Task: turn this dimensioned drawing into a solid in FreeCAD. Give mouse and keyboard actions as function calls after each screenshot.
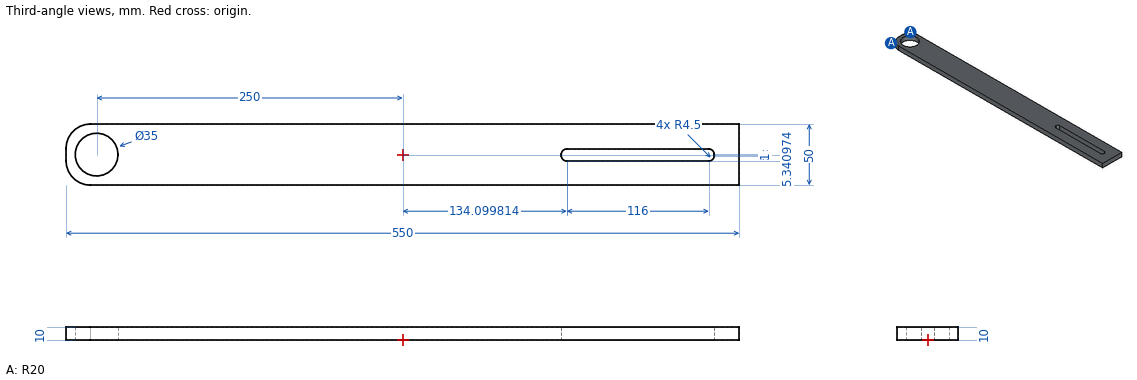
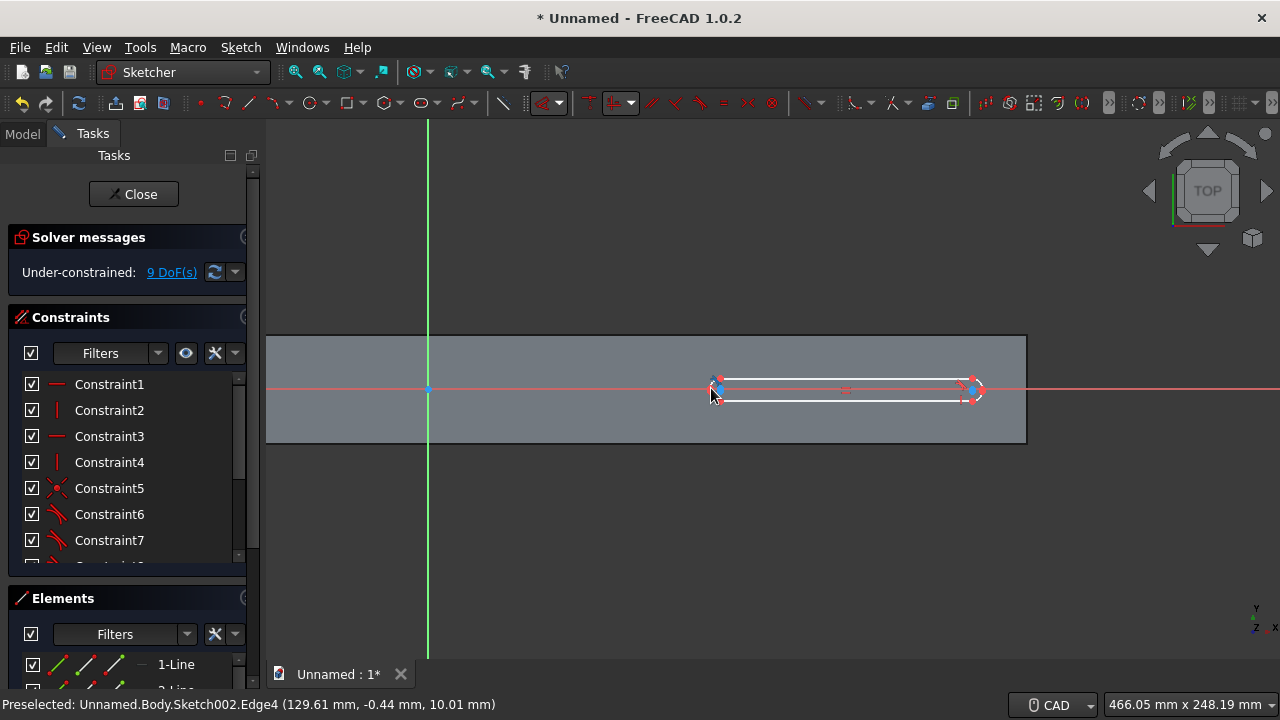
scroll(711, 396, up, 6)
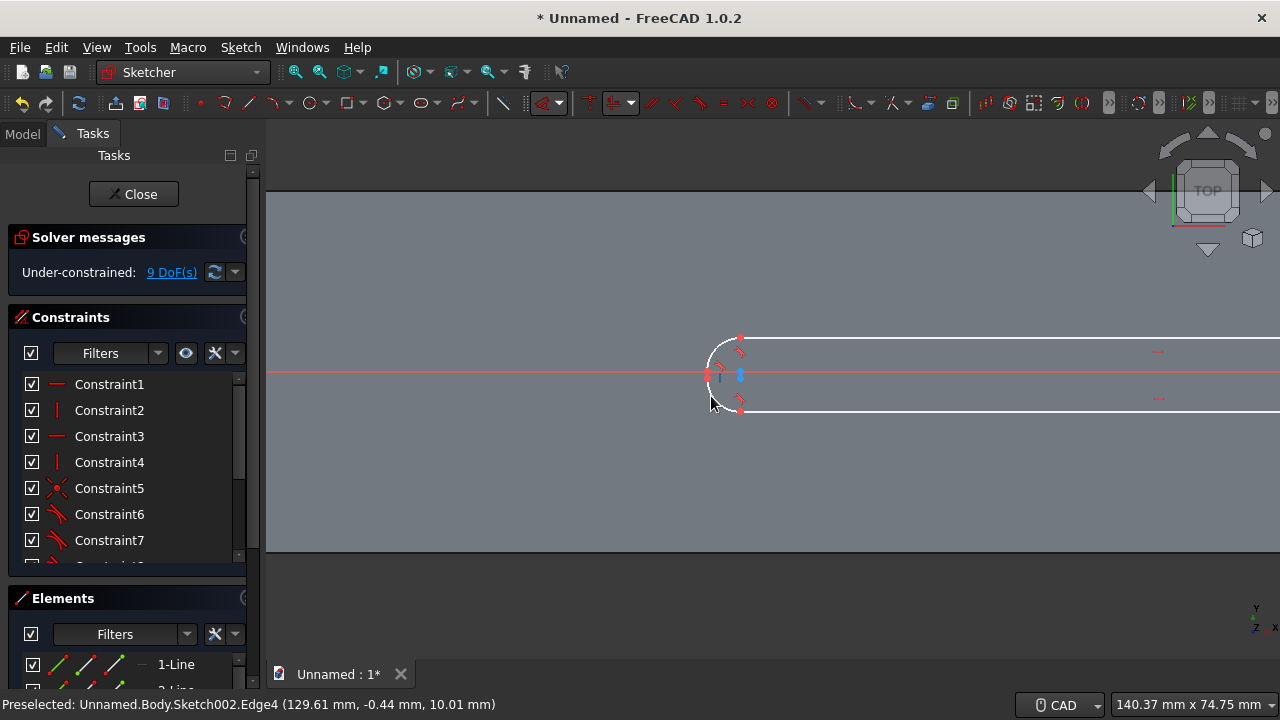
click(711, 394)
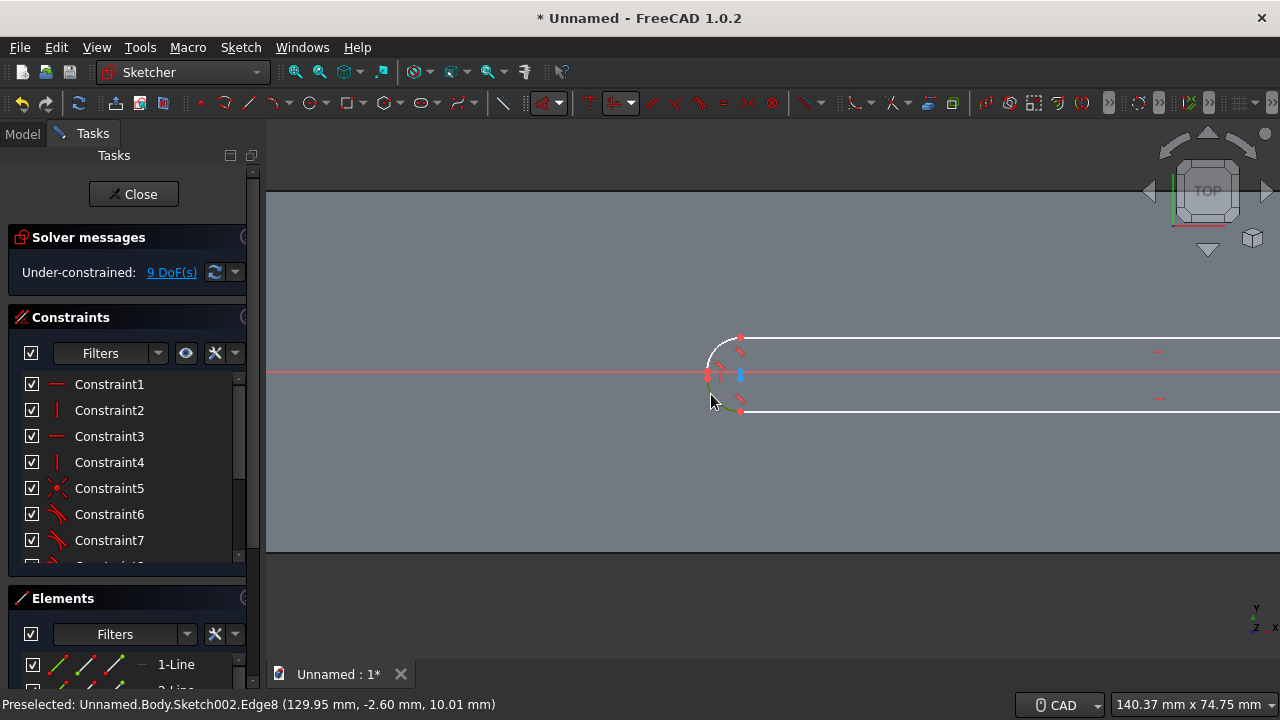
click(700, 104)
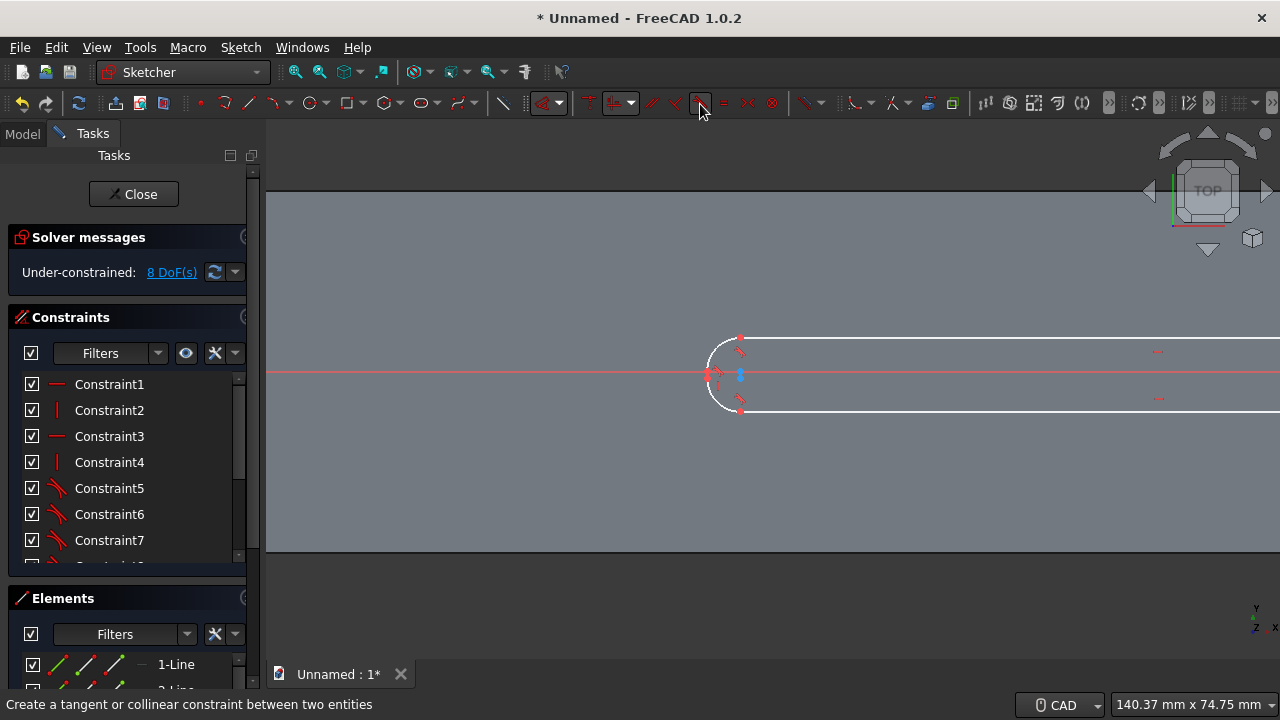
scroll(710, 395, down, 6)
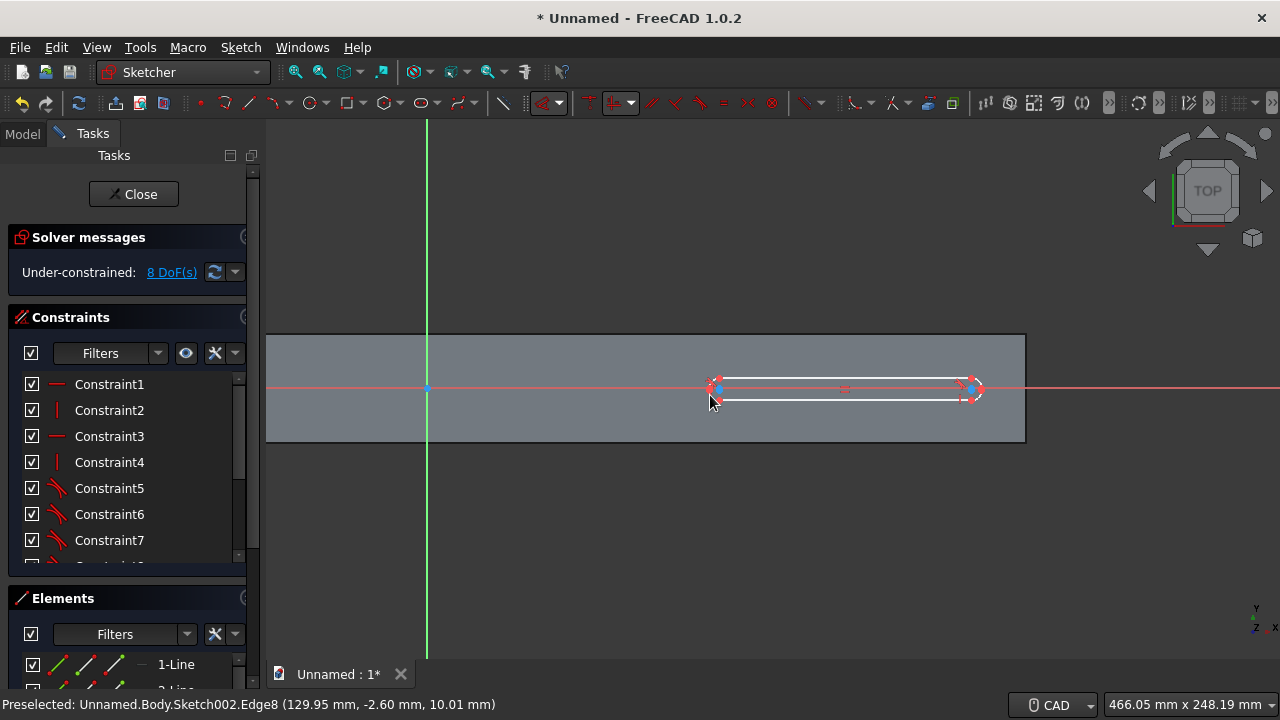
scroll(976, 399, up, 6)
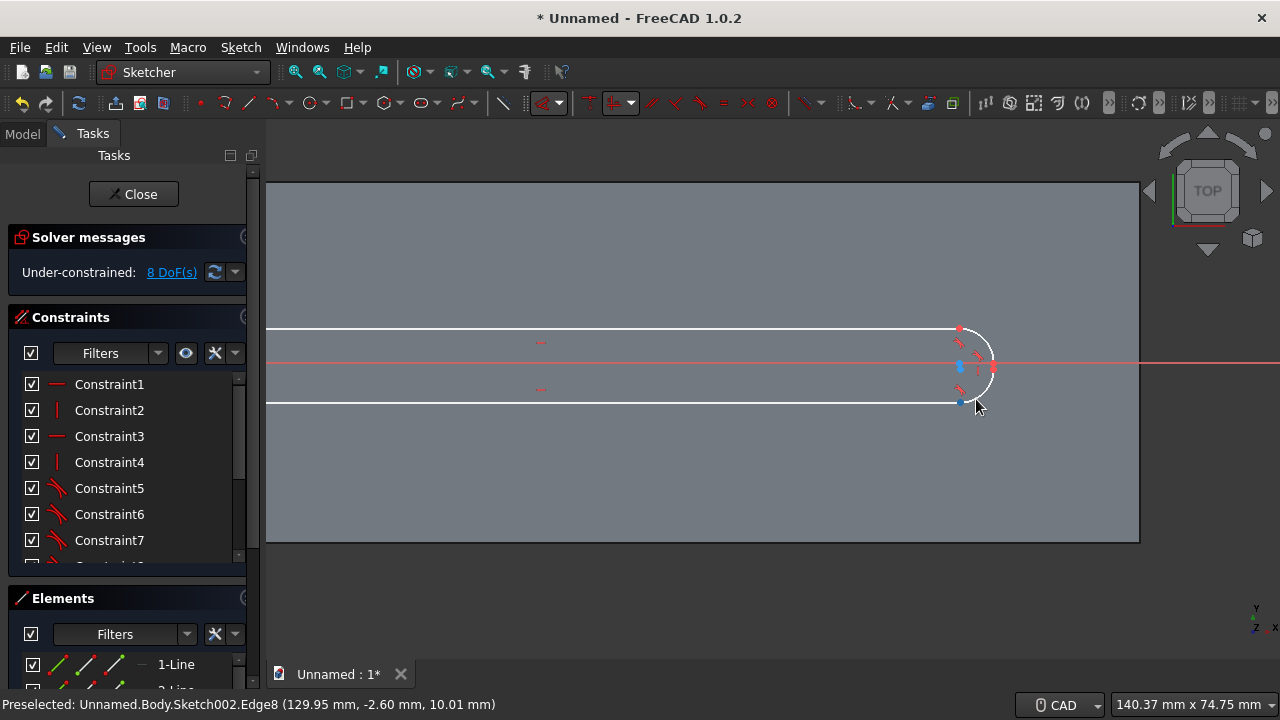
click(975, 399)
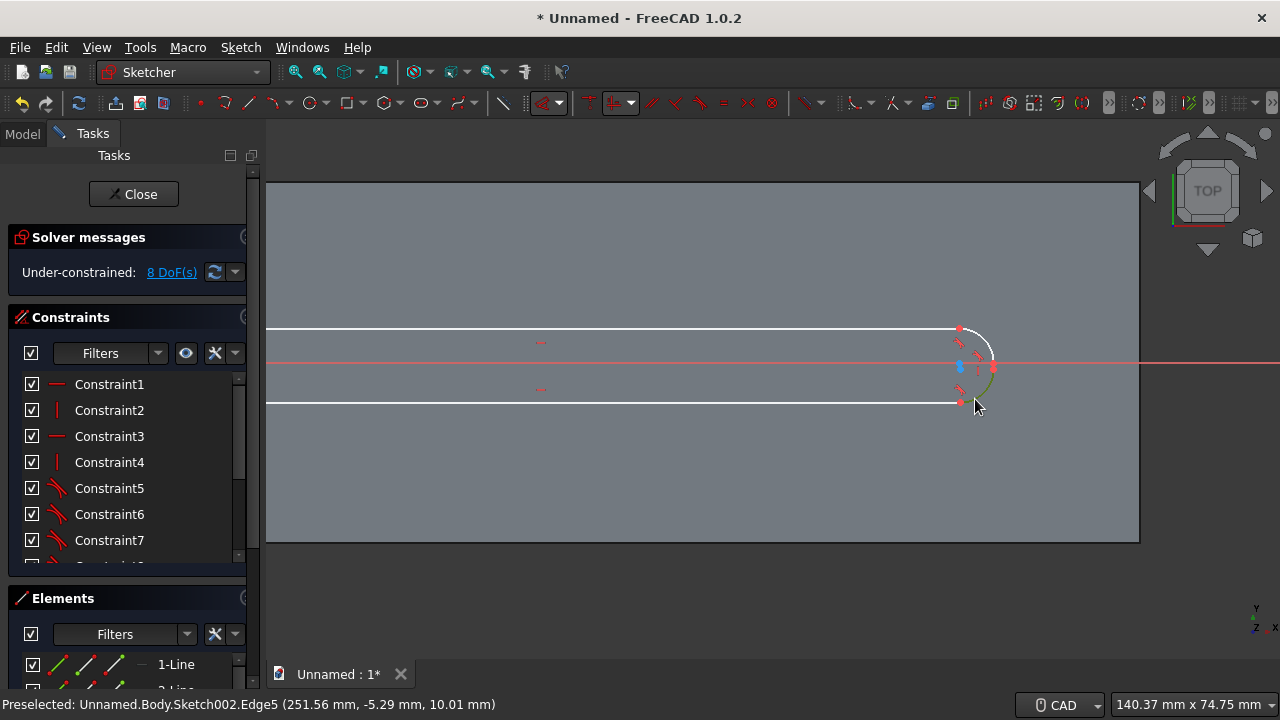
click(990, 347)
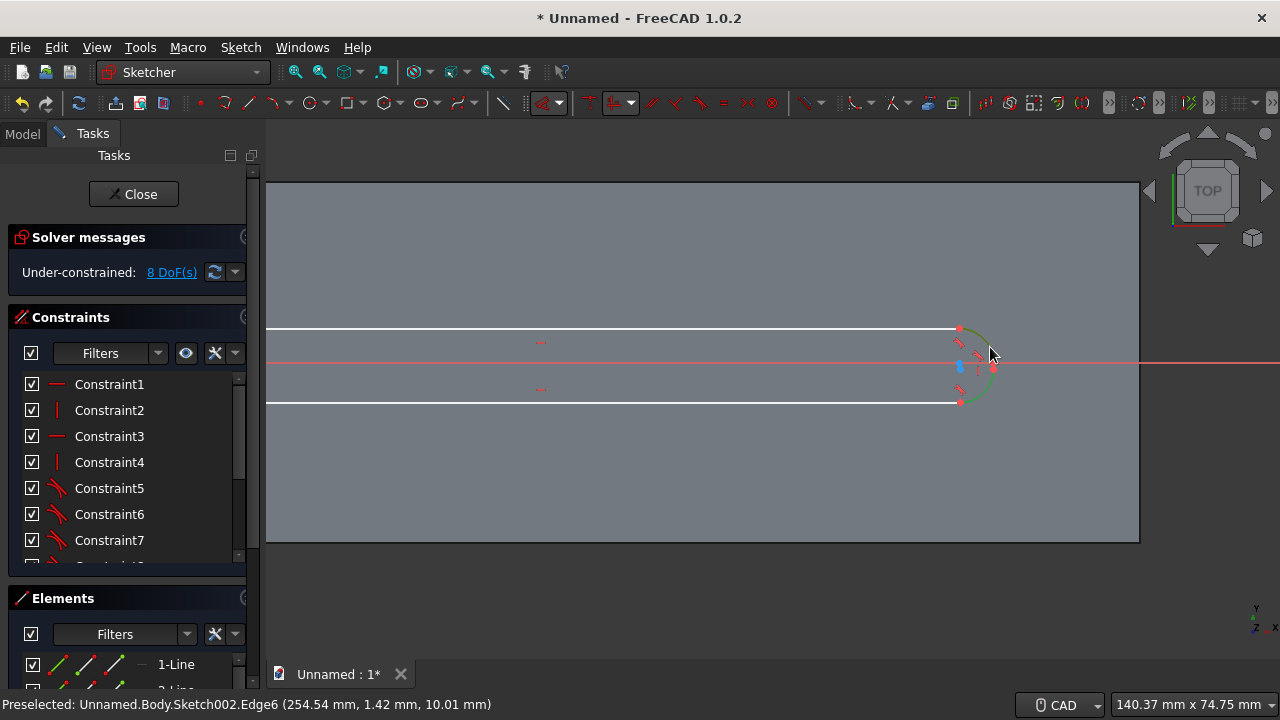
scroll(977, 399, down, 6)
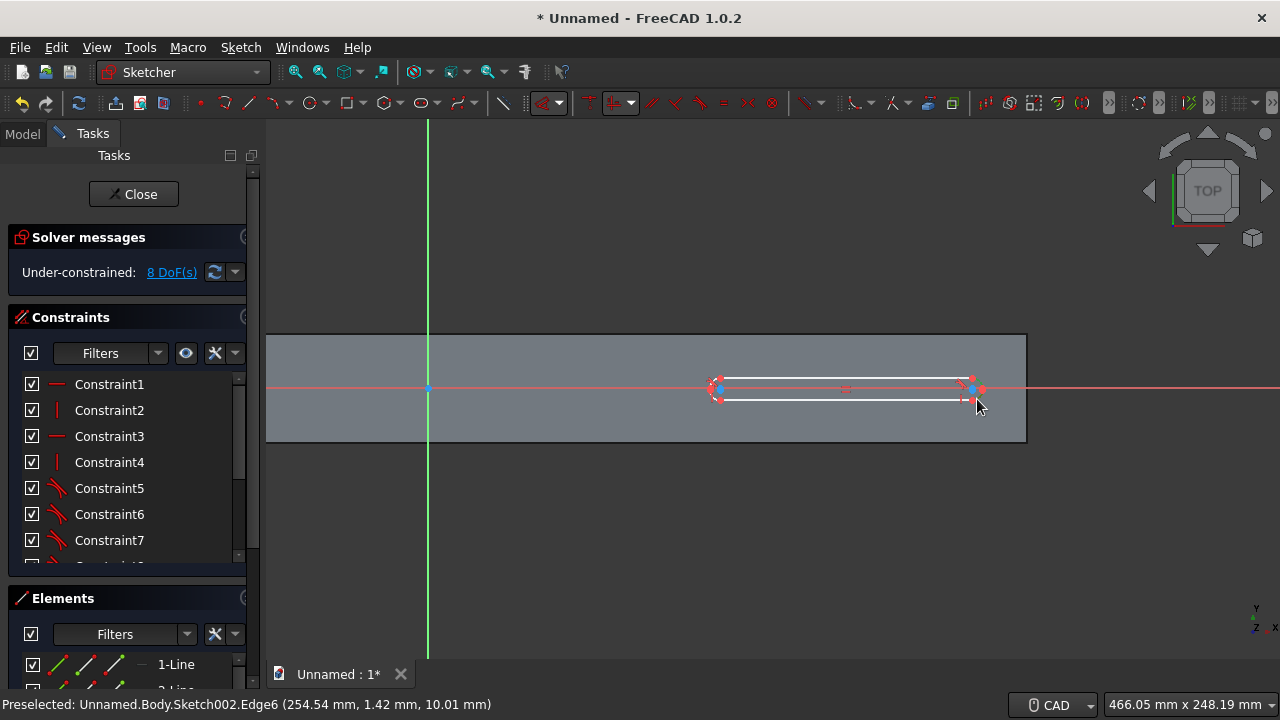
scroll(716, 379, up, 6)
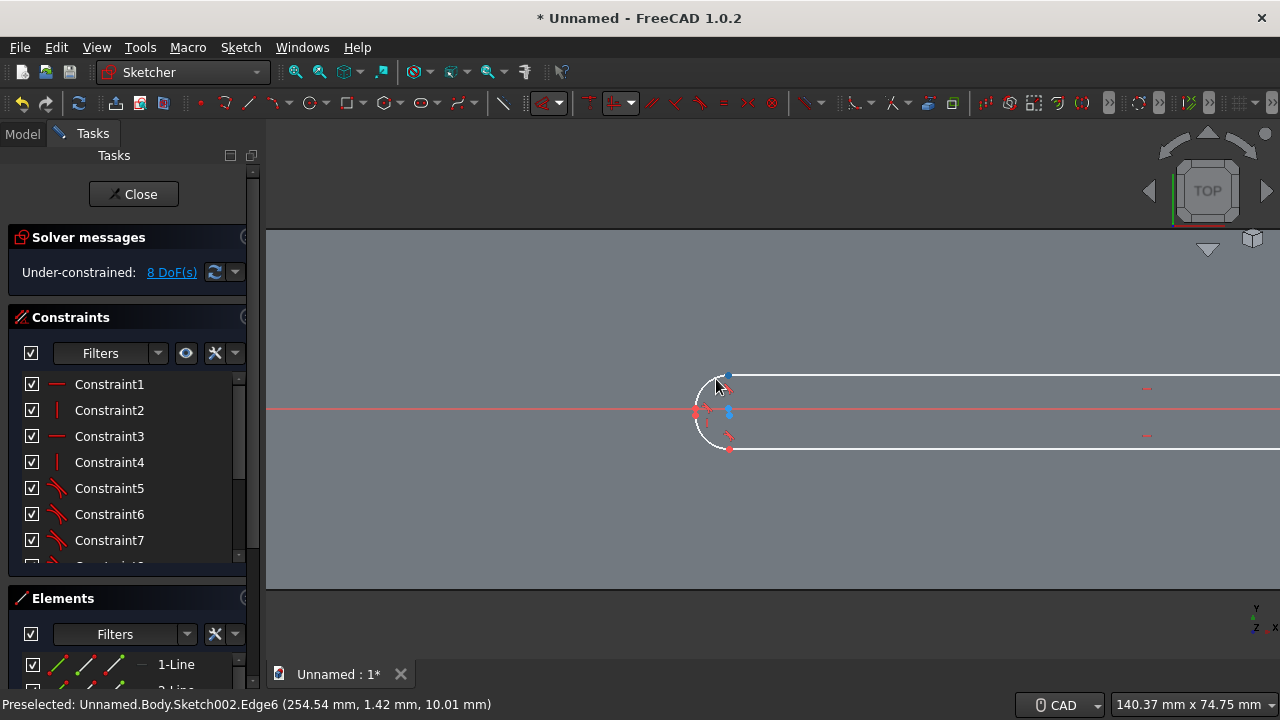
click(714, 379)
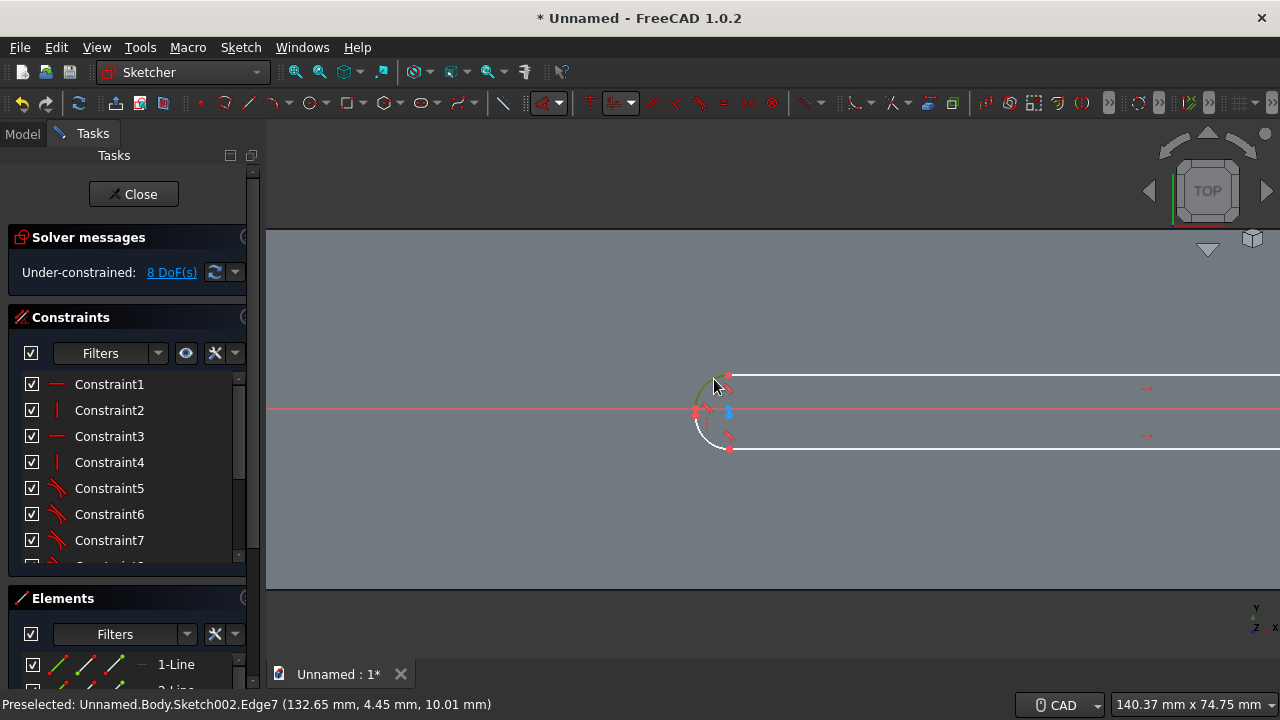
click(699, 431)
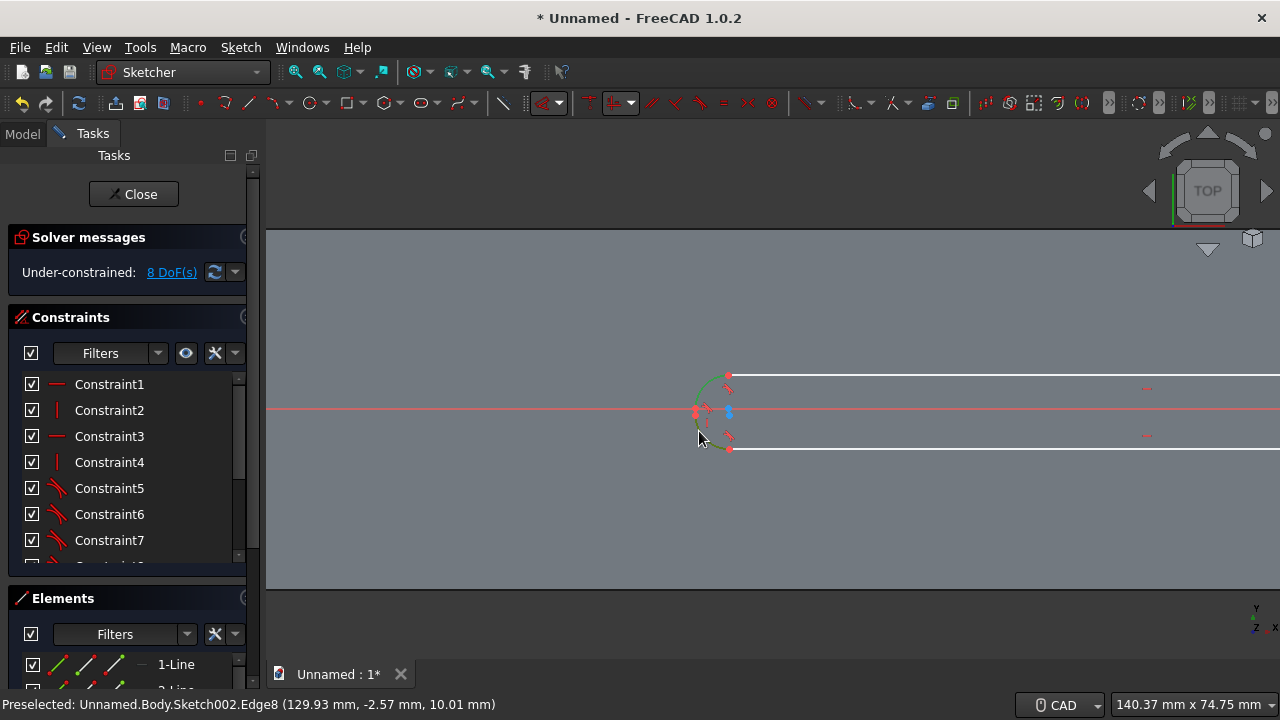
click(724, 104)